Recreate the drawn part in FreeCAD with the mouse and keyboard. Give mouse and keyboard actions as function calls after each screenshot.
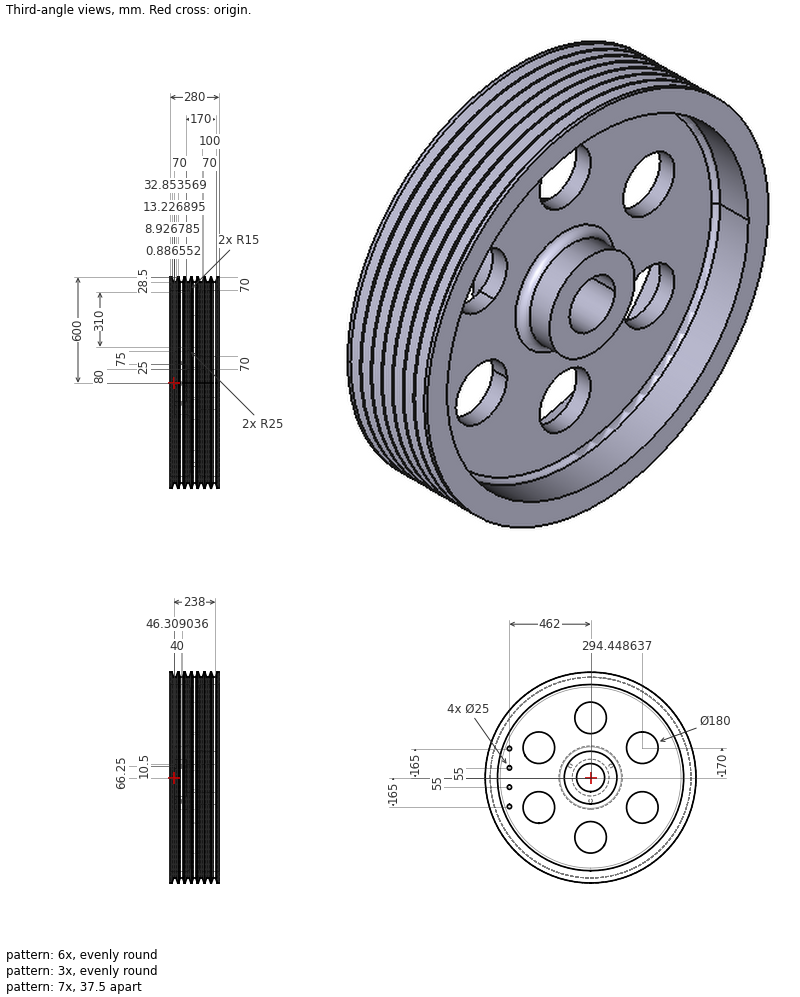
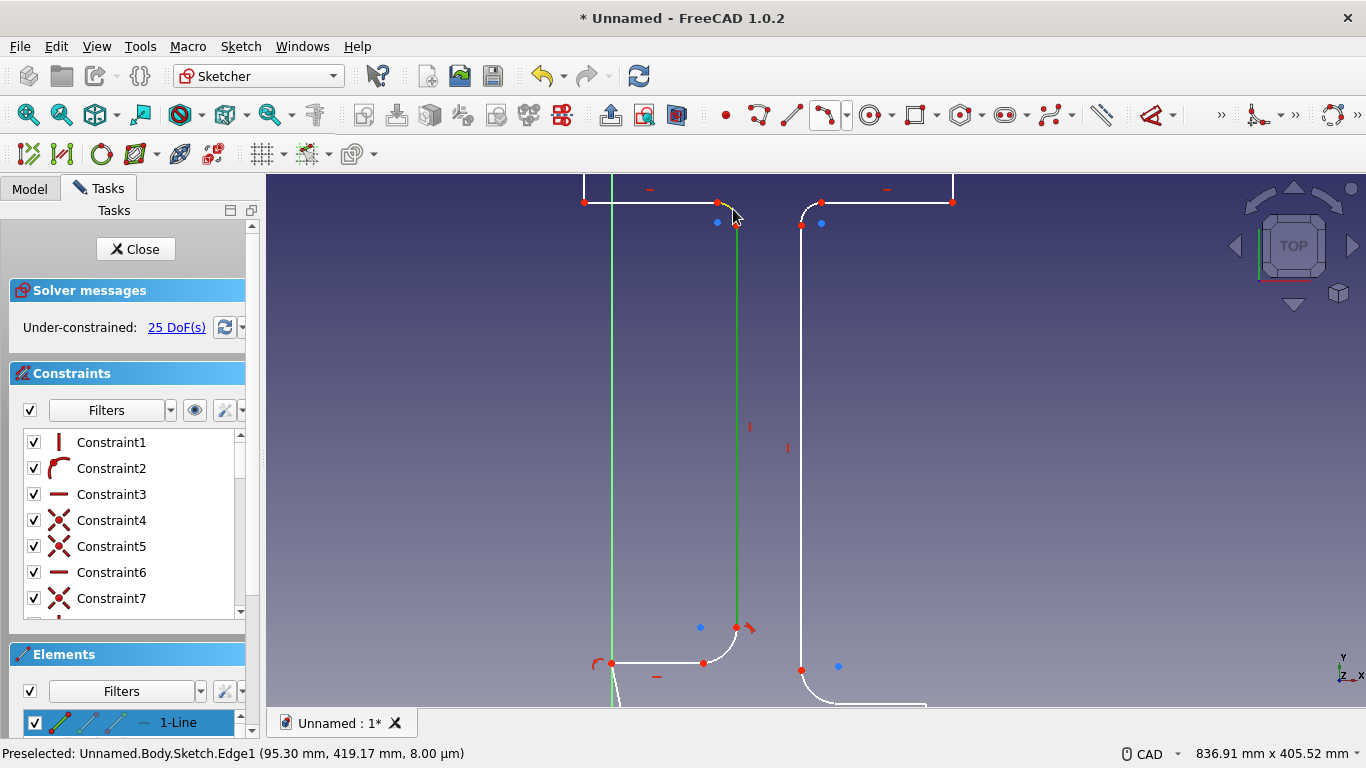
click(732, 210)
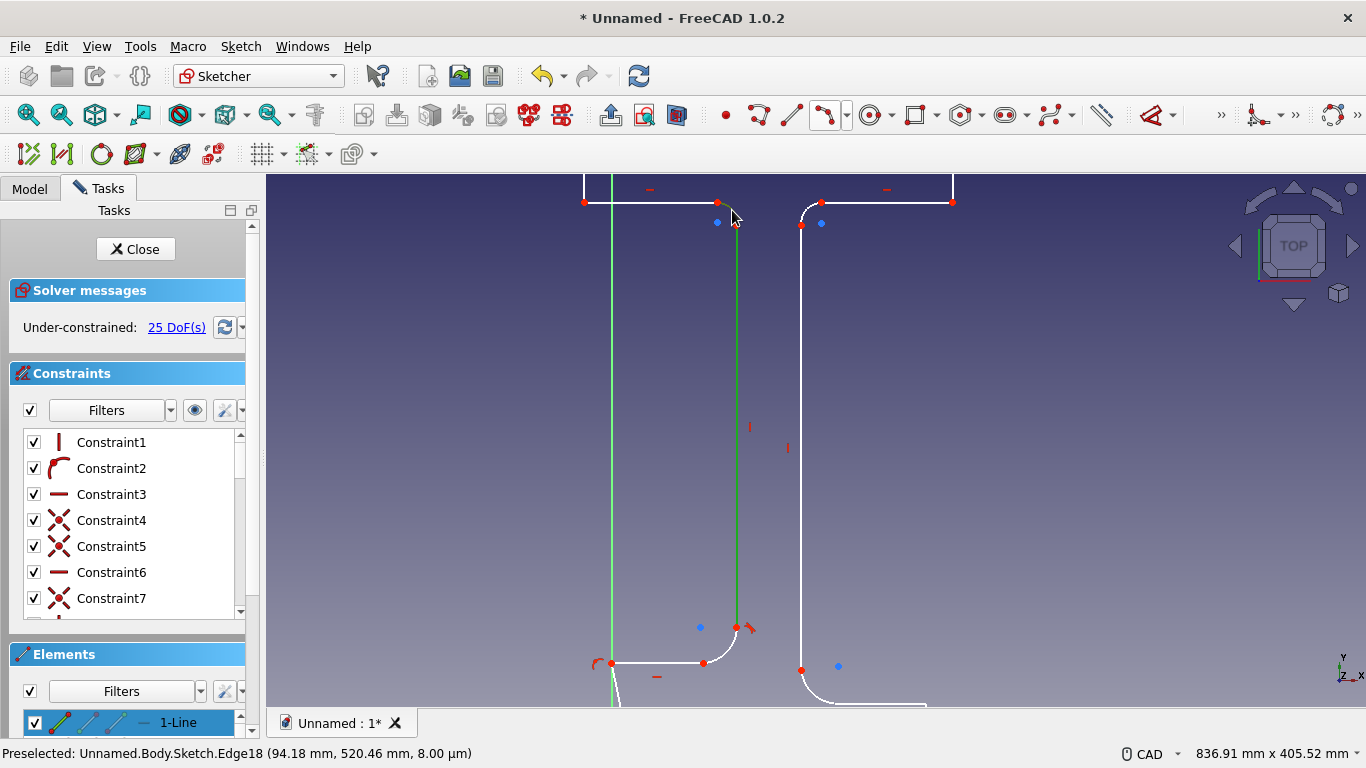
key(t)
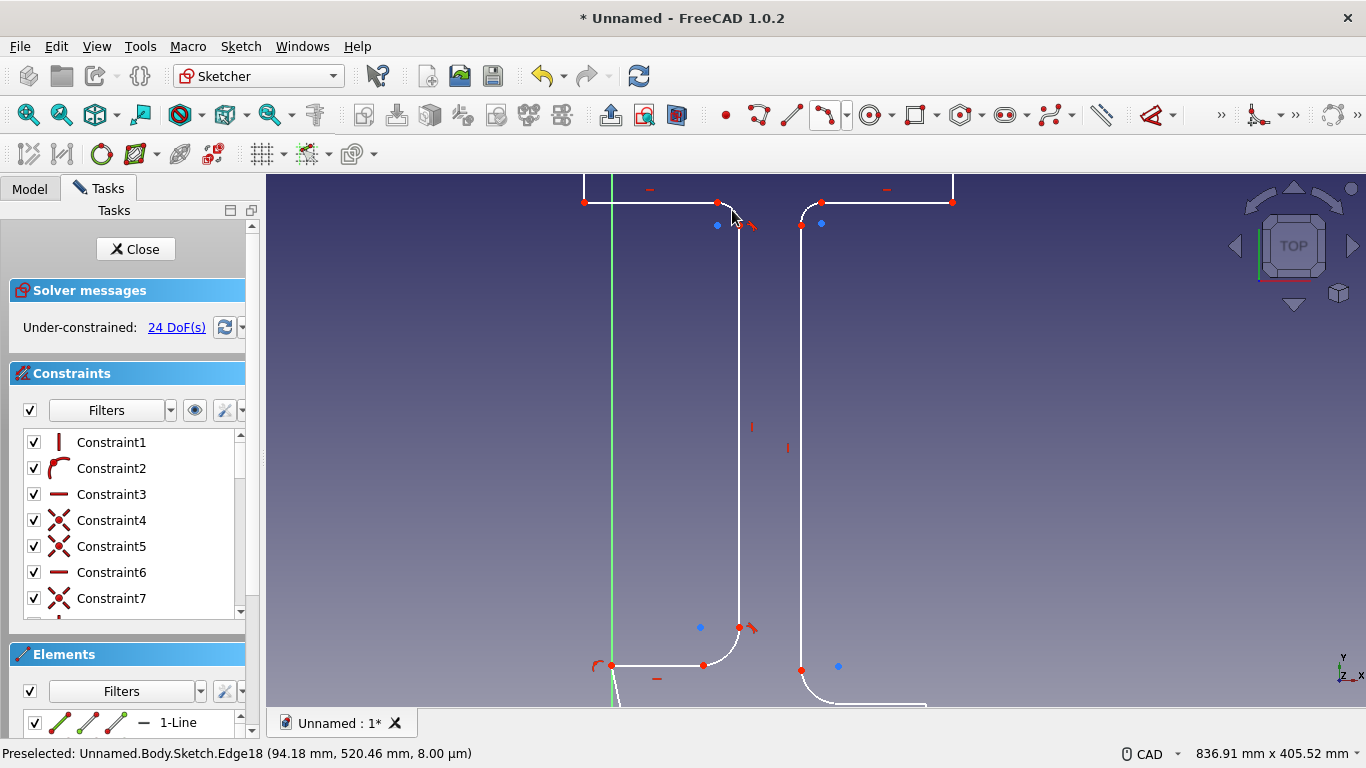
click(676, 666)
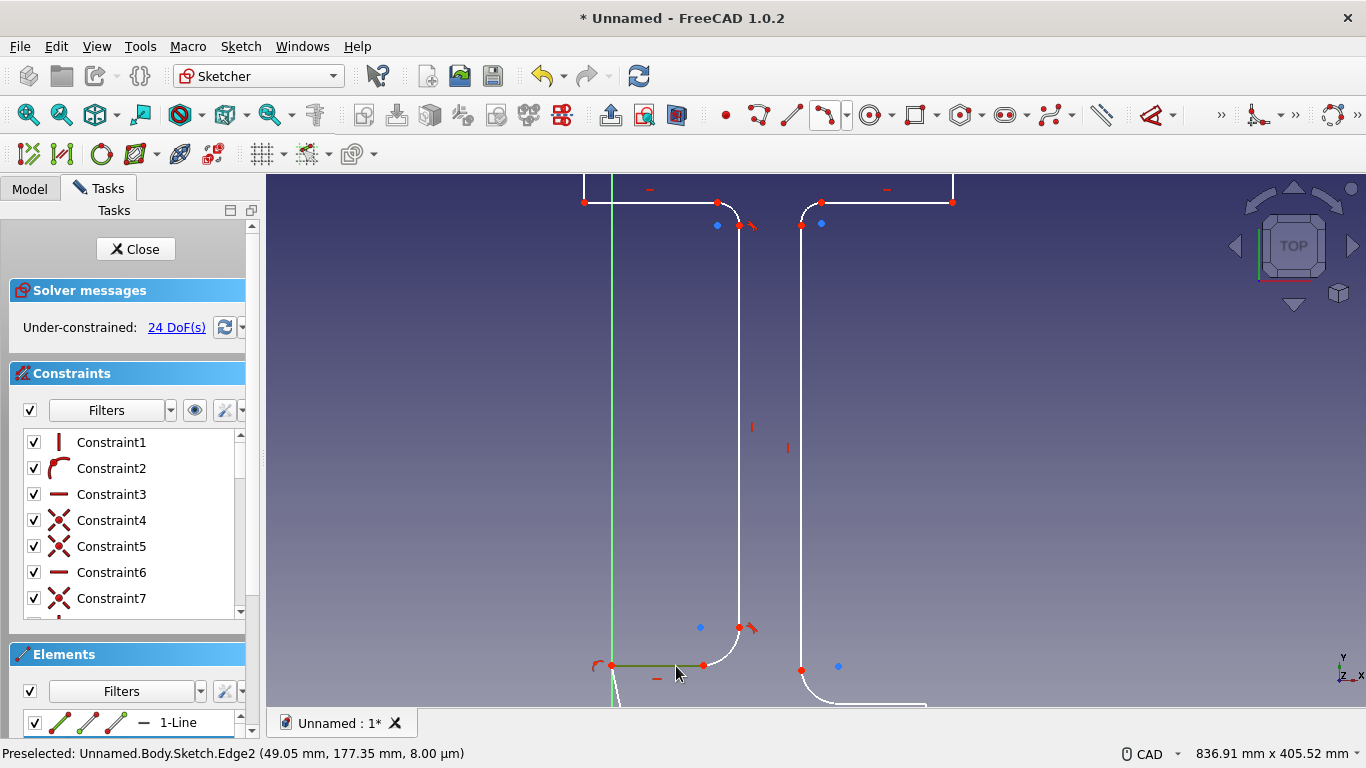
click(720, 661)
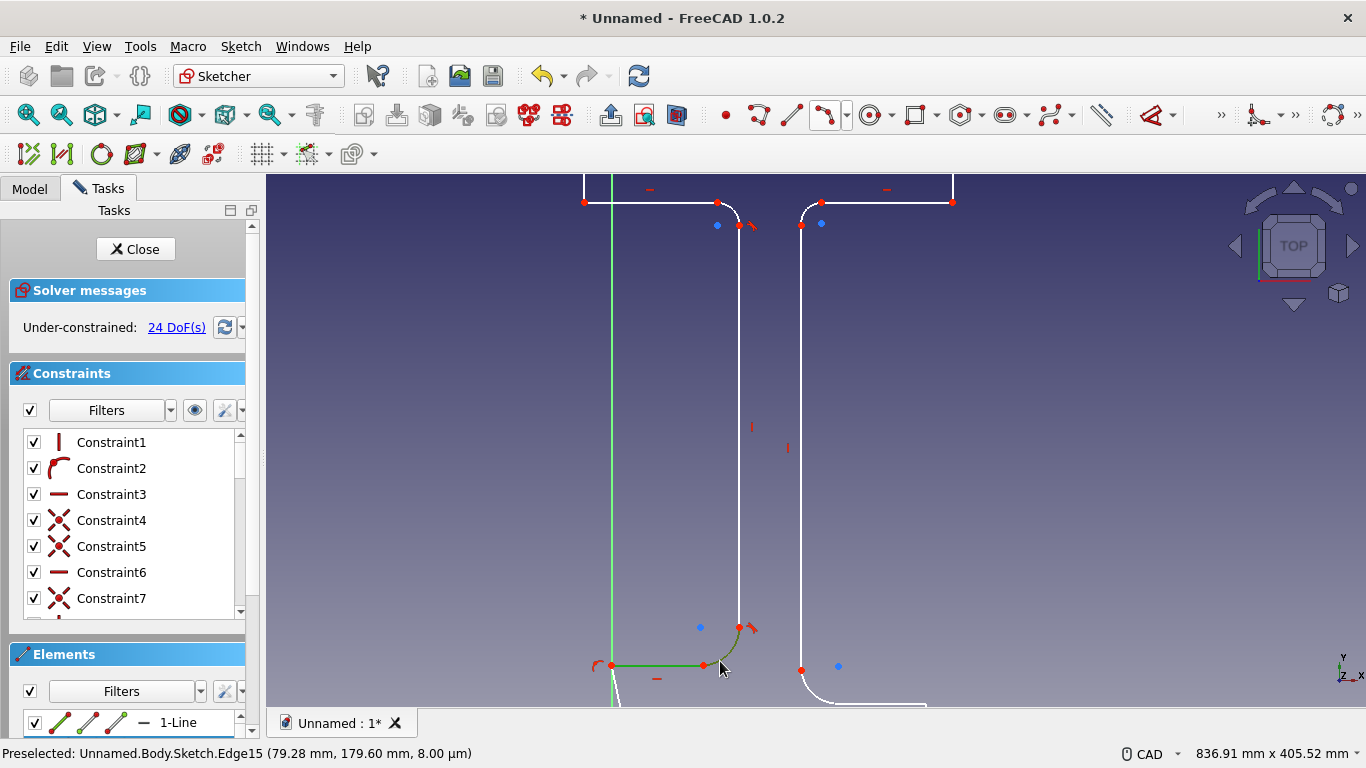
key(t)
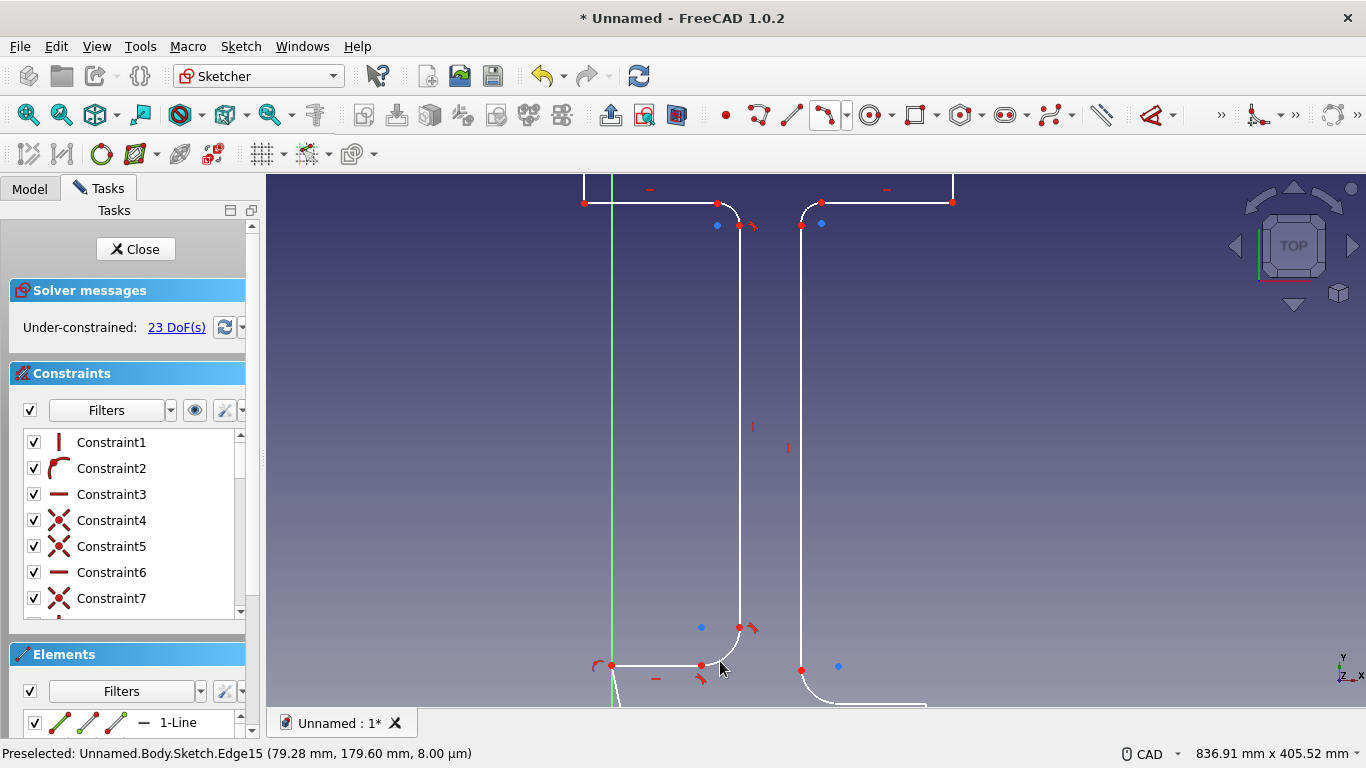
scroll(730, 388, down, 4)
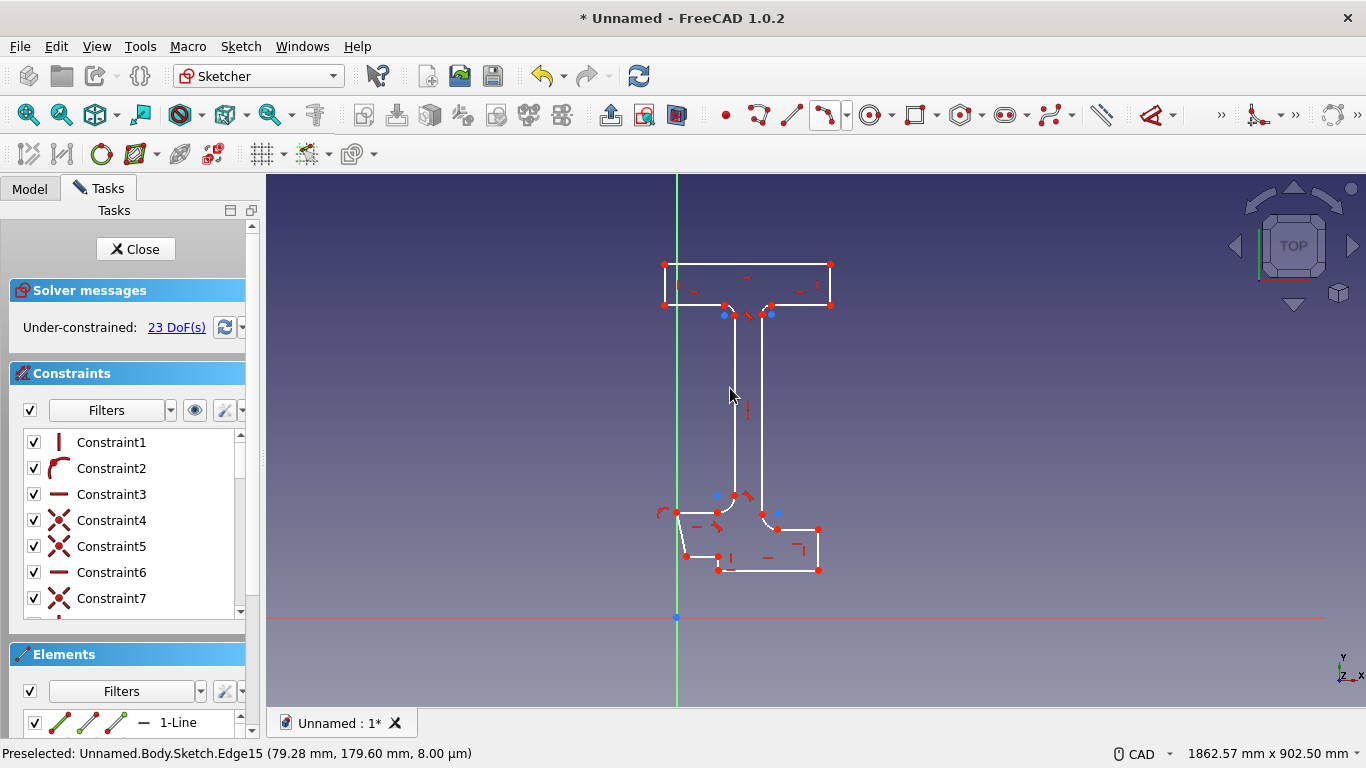
click(806, 530)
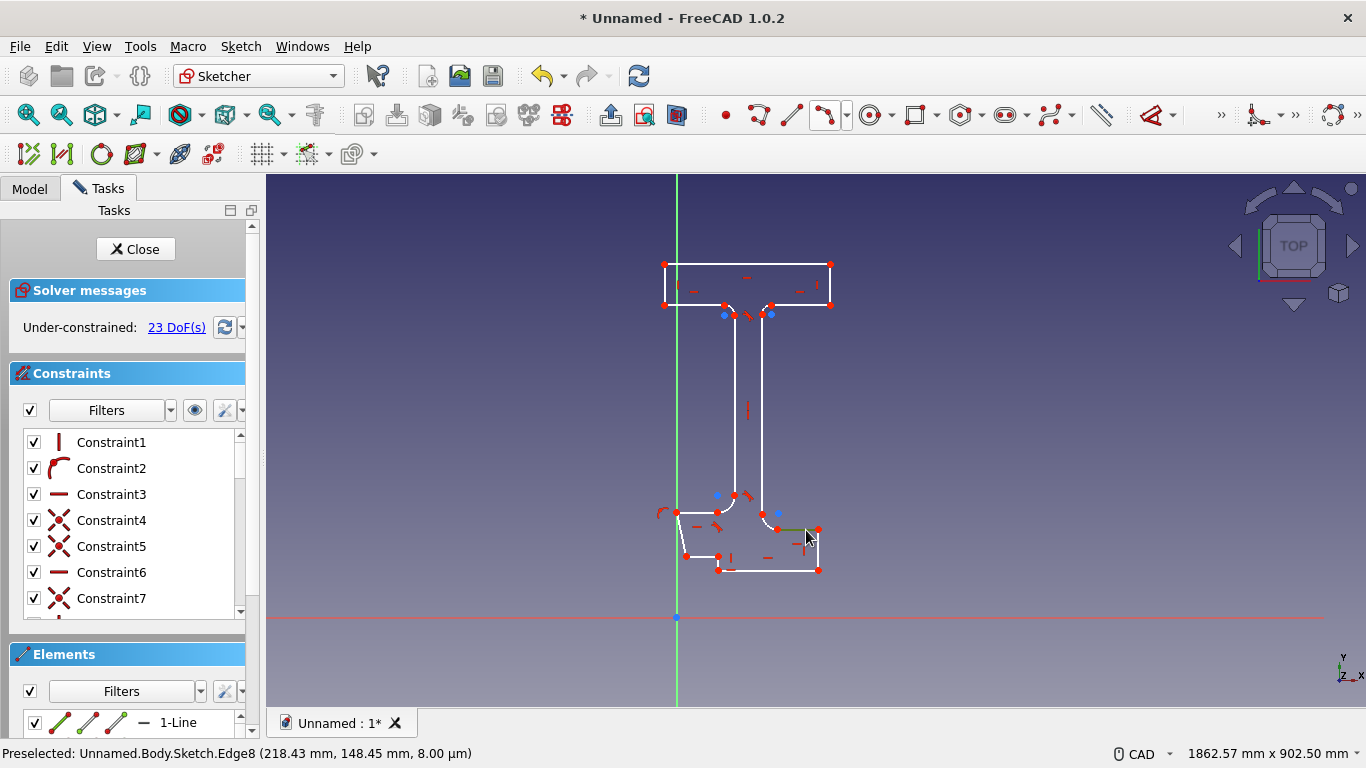
scroll(767, 525, up, 2)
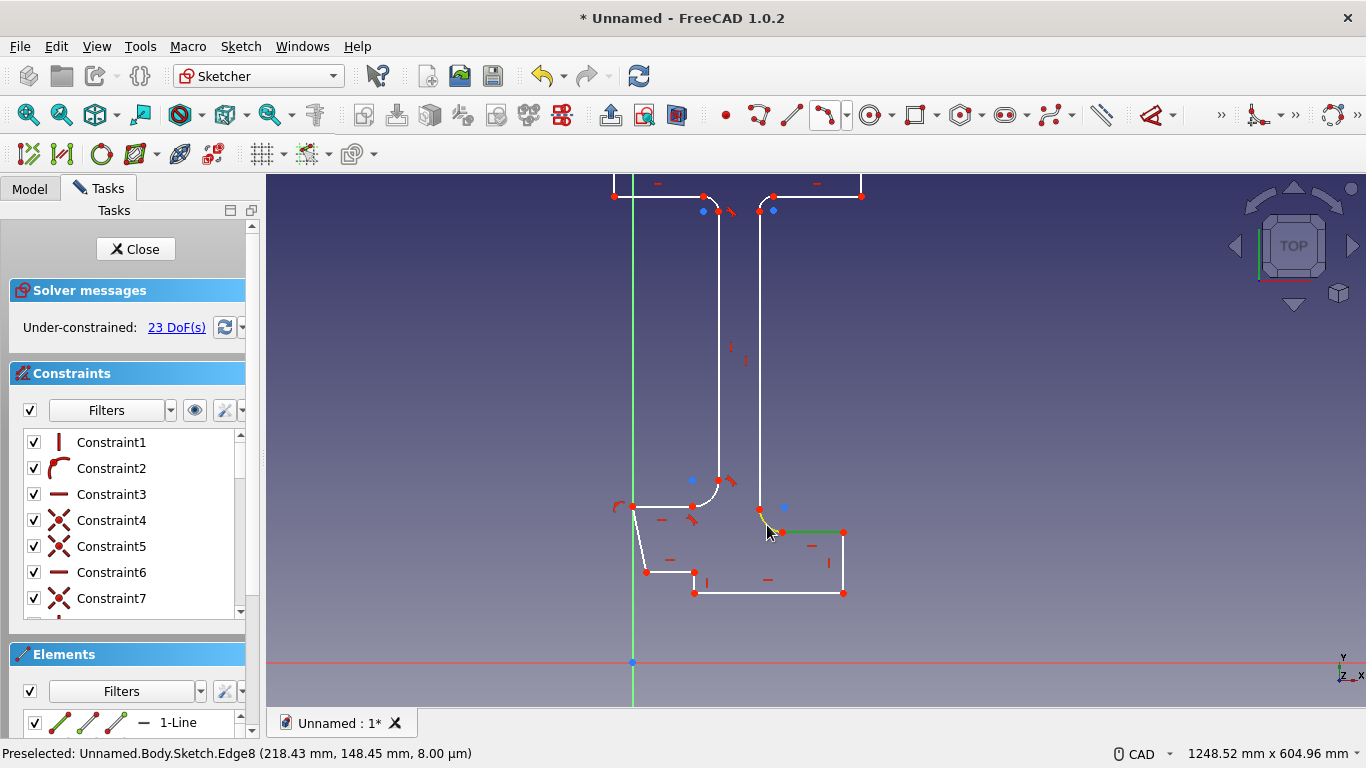
click(767, 525)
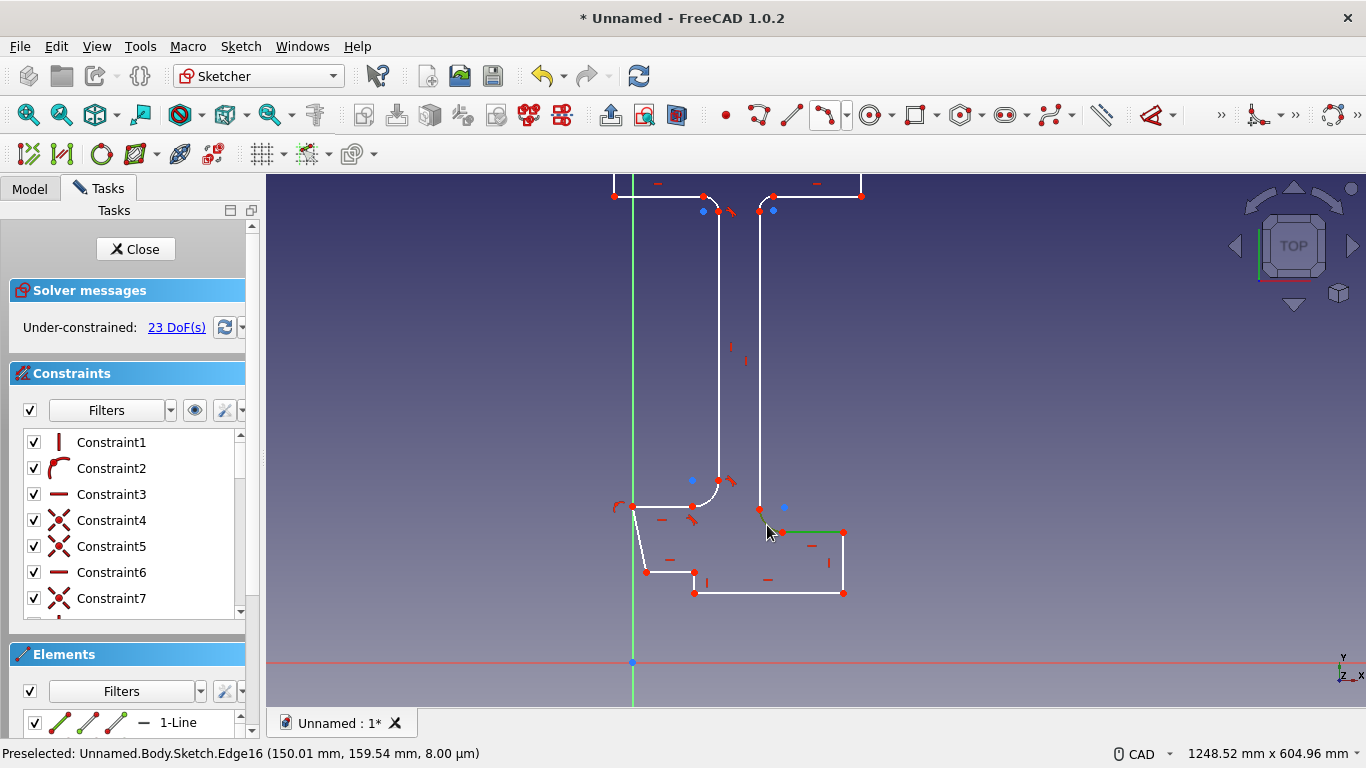
key(t)